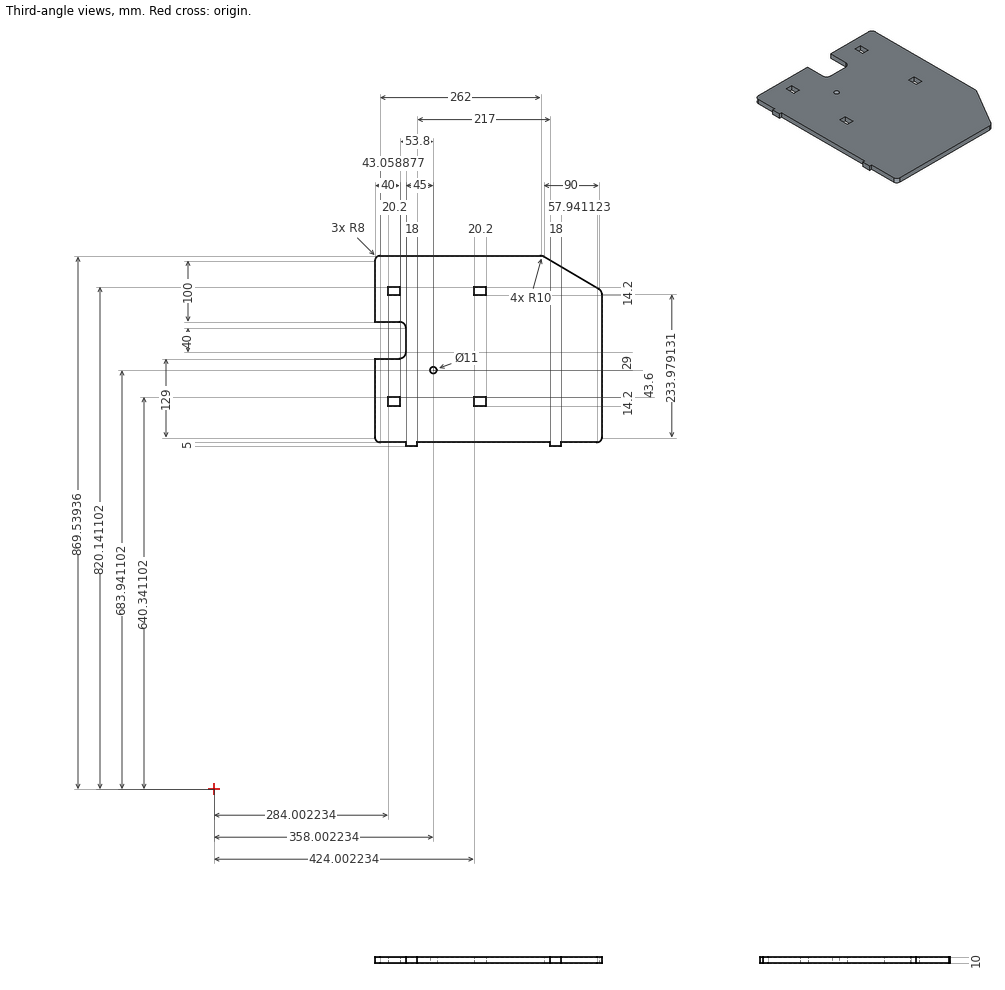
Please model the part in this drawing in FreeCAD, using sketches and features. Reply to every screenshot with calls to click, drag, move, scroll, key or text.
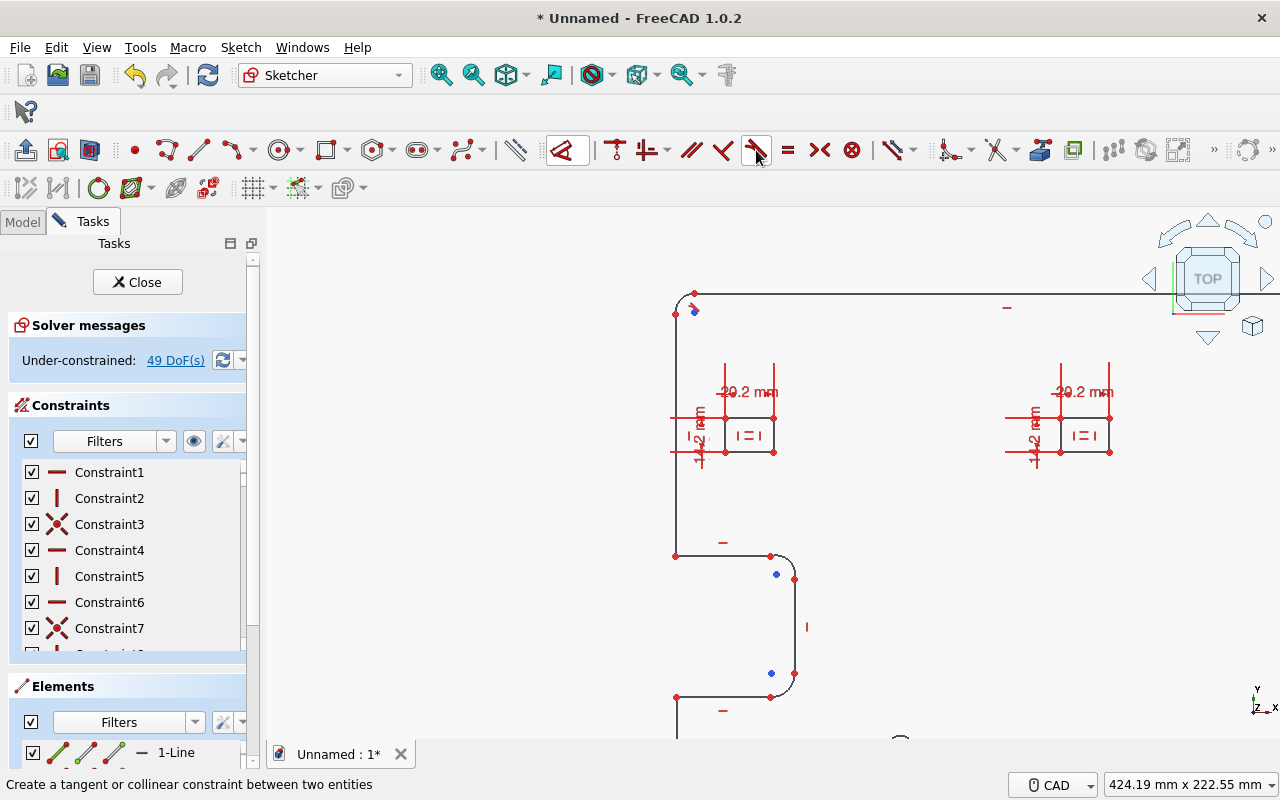
scroll(685, 302, down, 9)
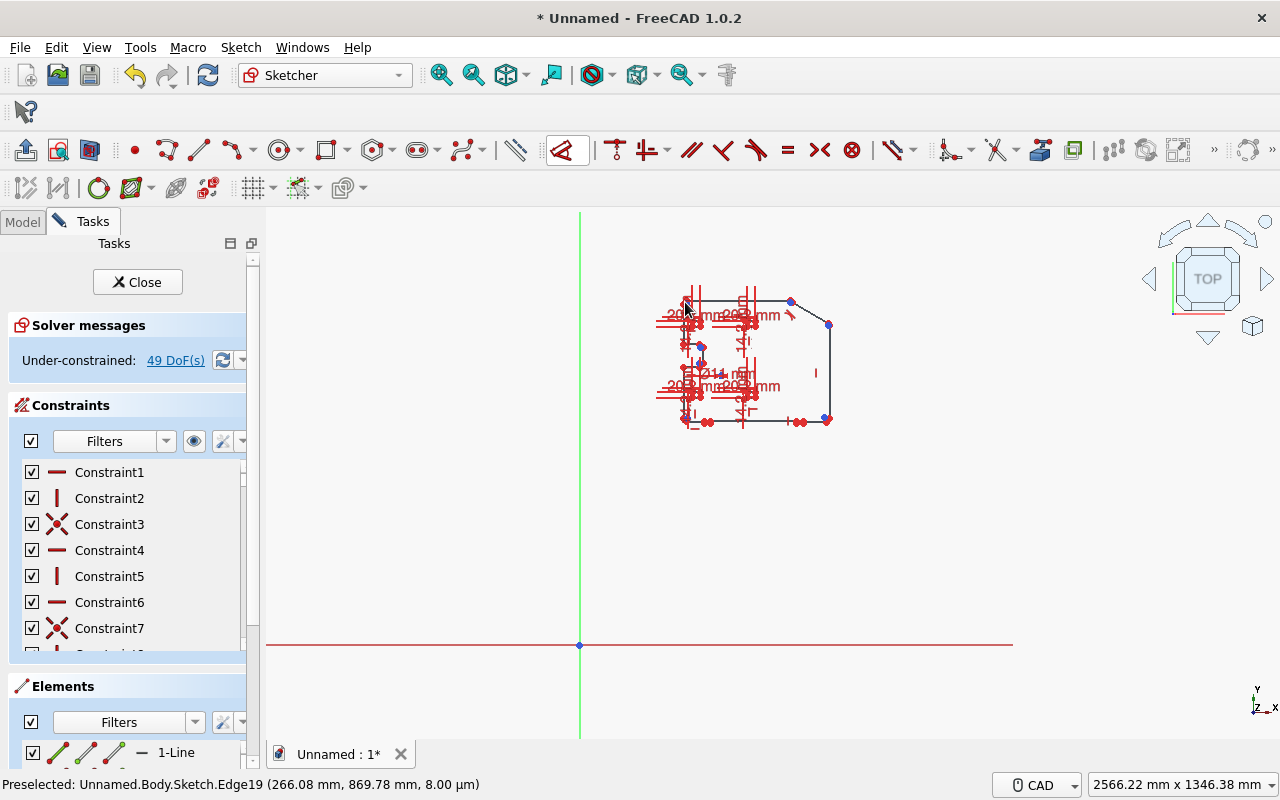
scroll(684, 316, up, 2)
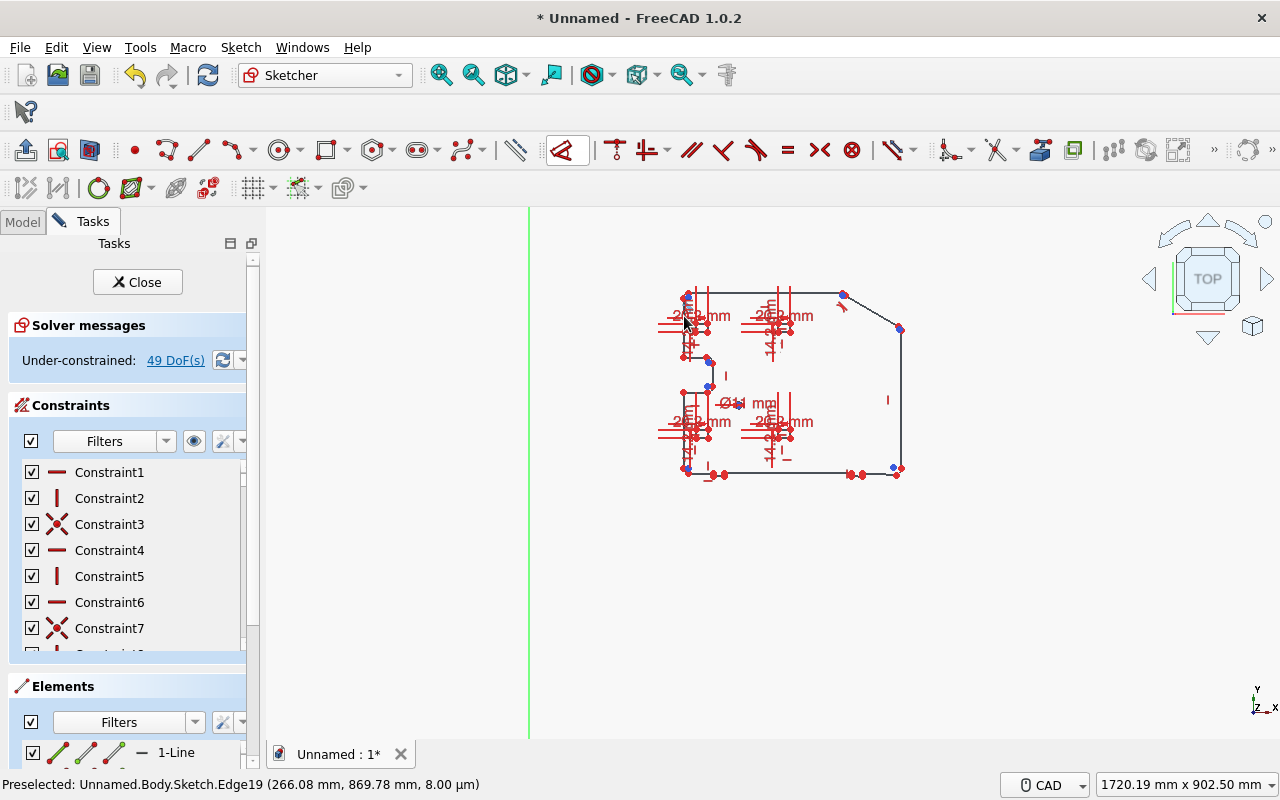
scroll(684, 316, up, 4)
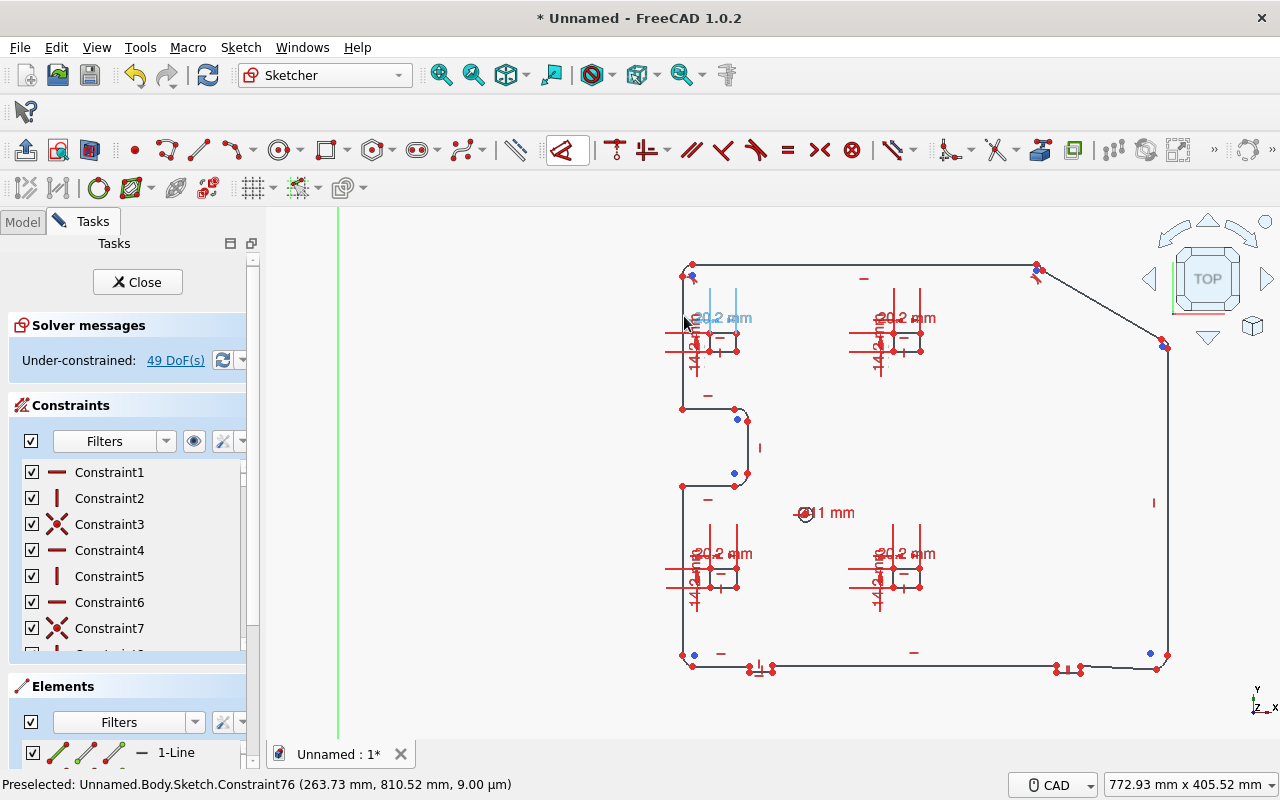
click(683, 316)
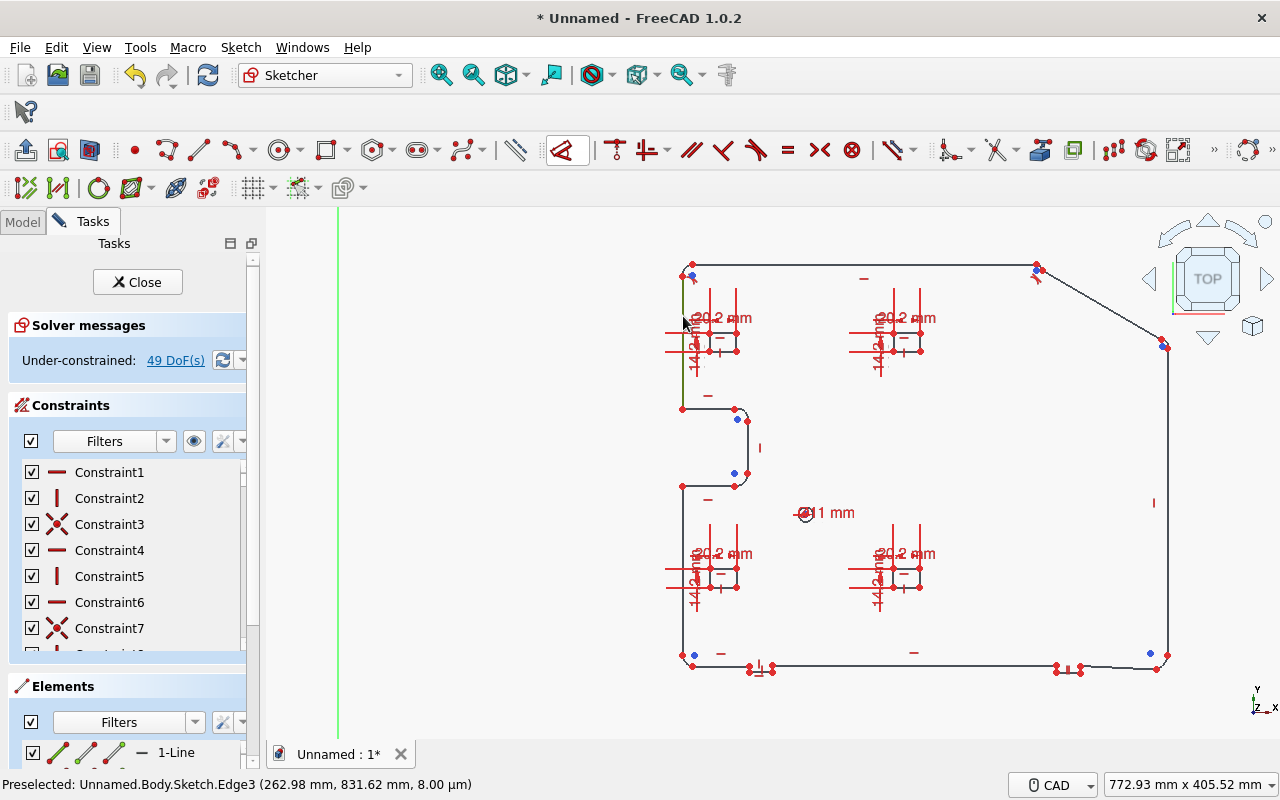
scroll(685, 268, up, 3)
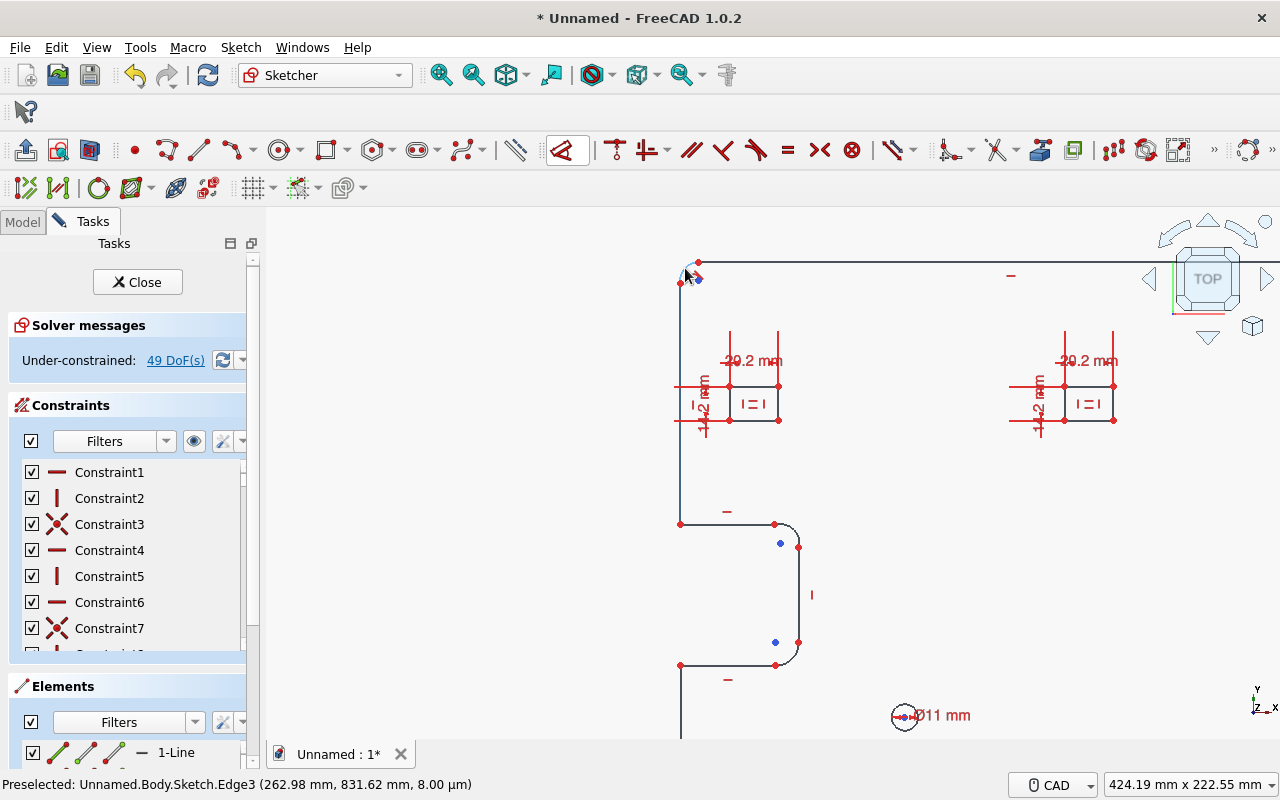
click(685, 269)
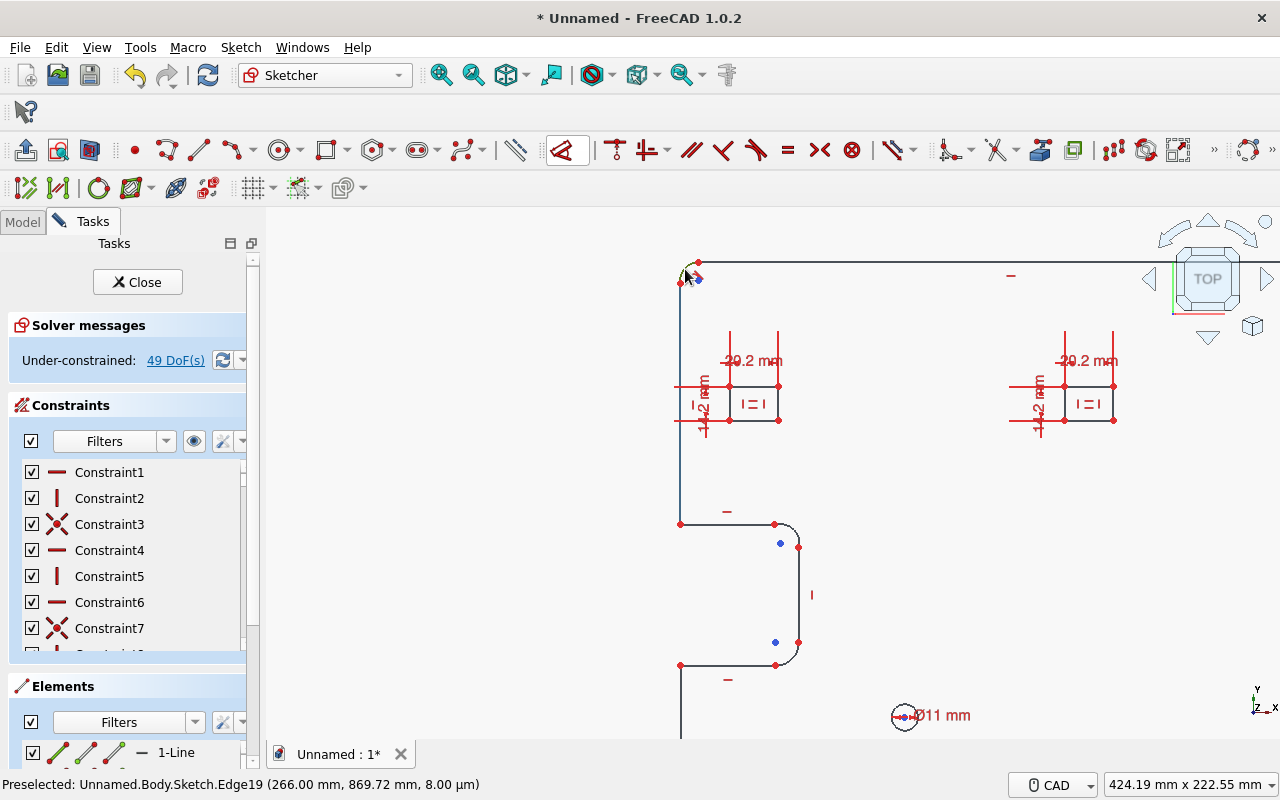
click(756, 150)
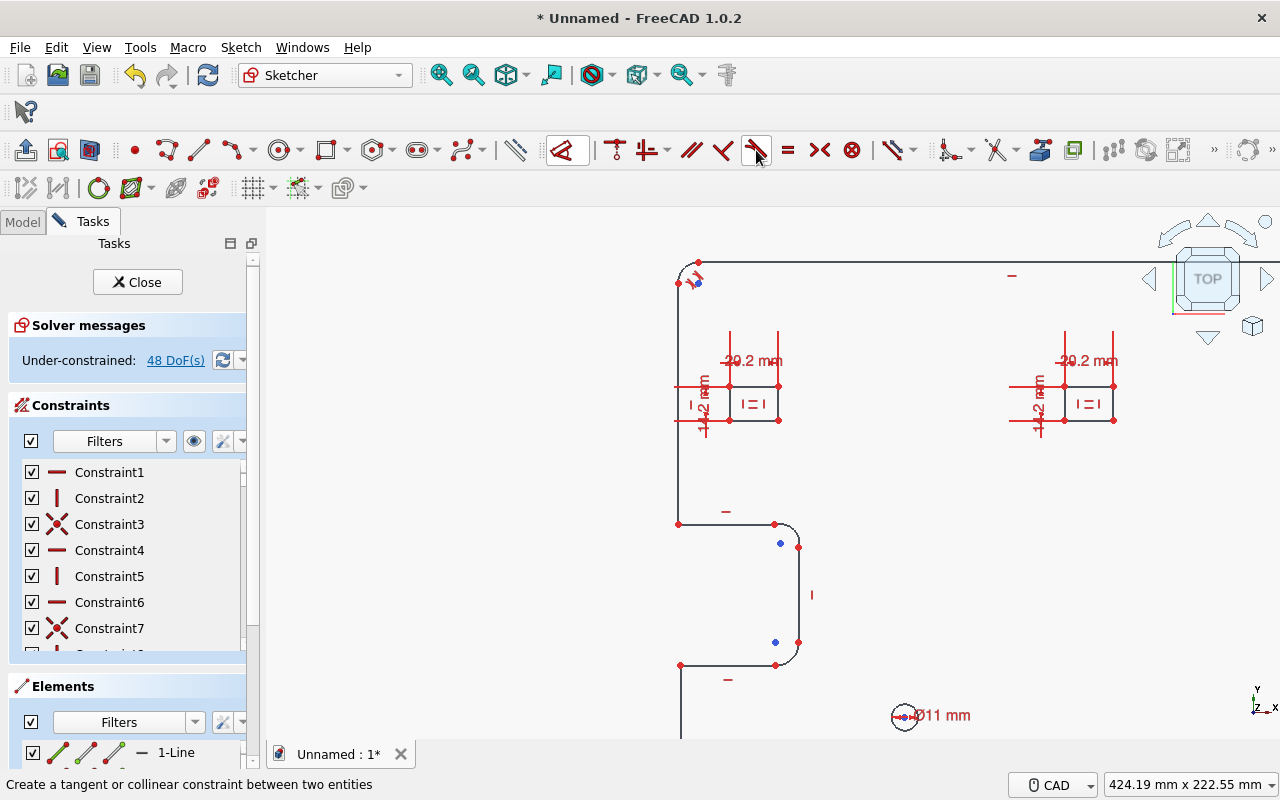
click(707, 525)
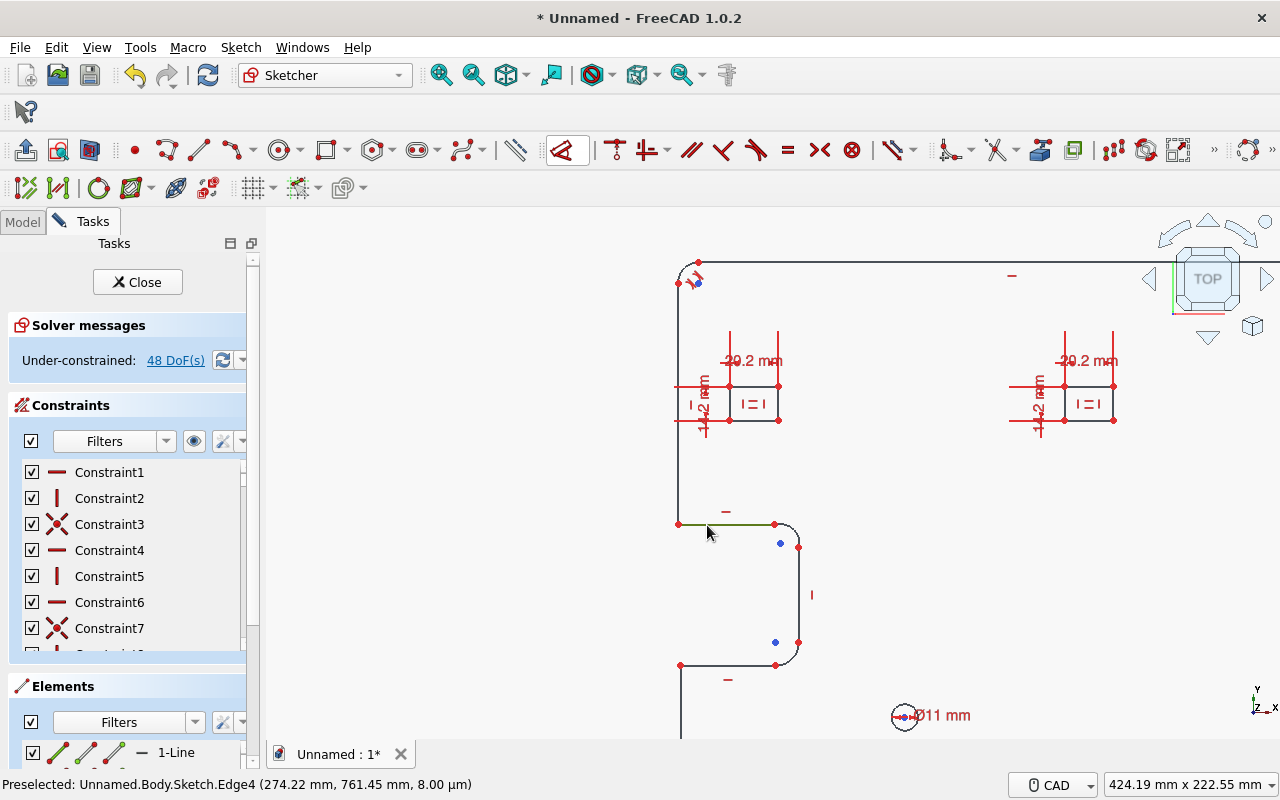
click(798, 536)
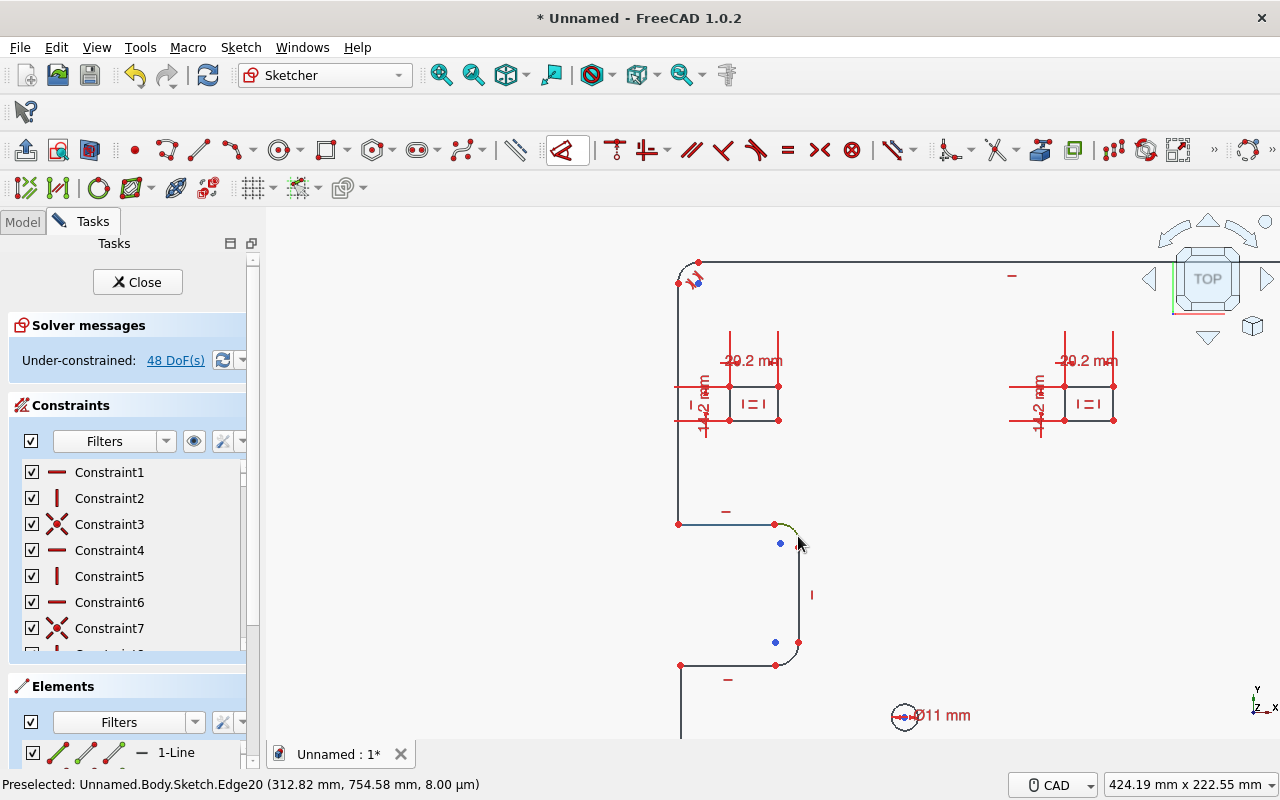
key(t)